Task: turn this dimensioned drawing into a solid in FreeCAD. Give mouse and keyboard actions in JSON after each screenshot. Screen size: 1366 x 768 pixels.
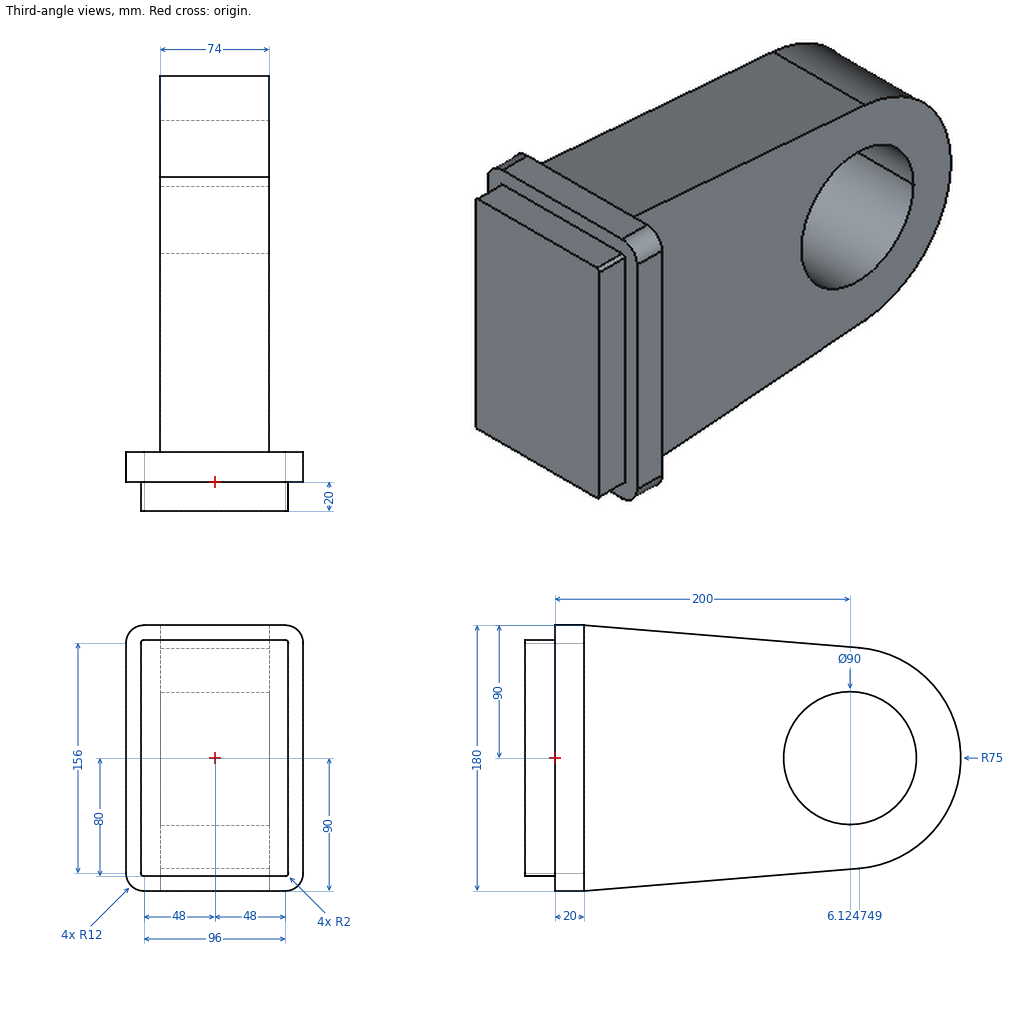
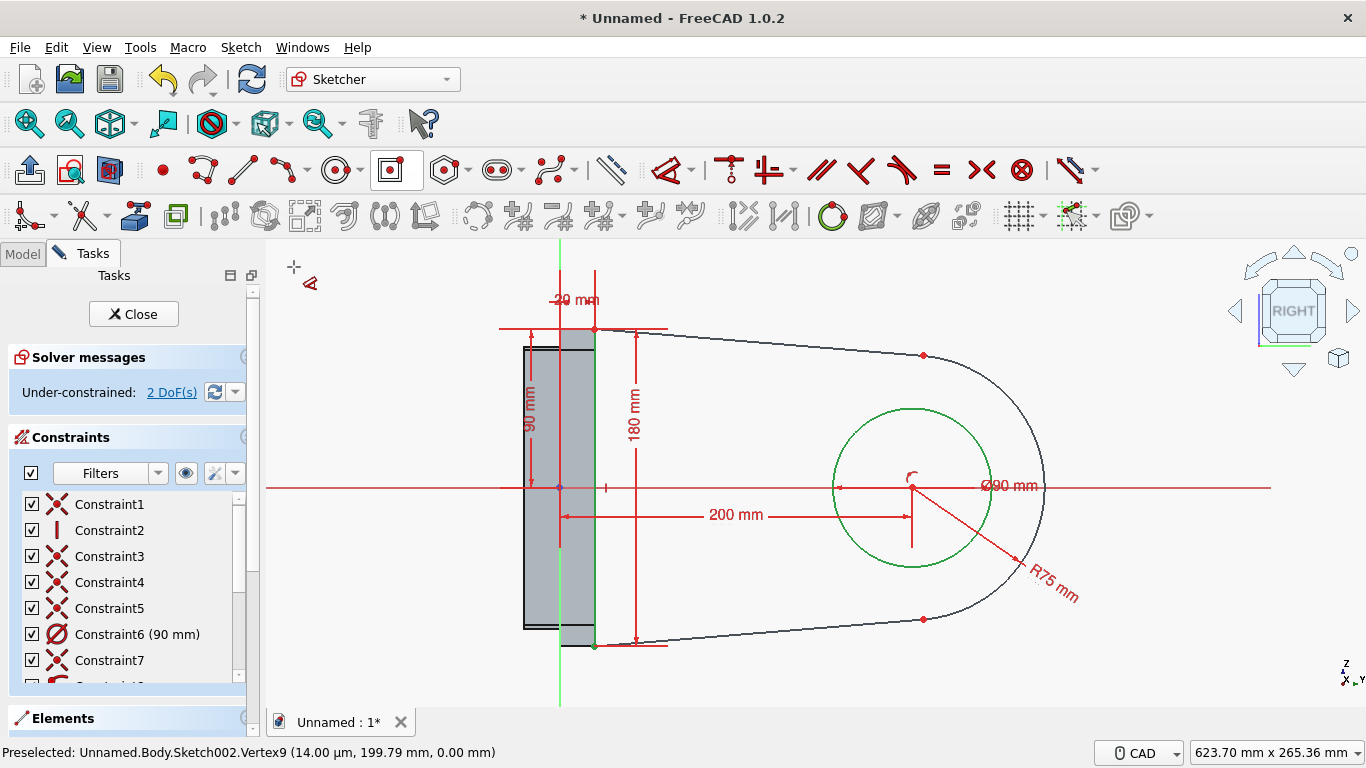
{"action": "scroll", "coordinate": [924, 620], "scroll_direction": "up", "scroll_amount": 7}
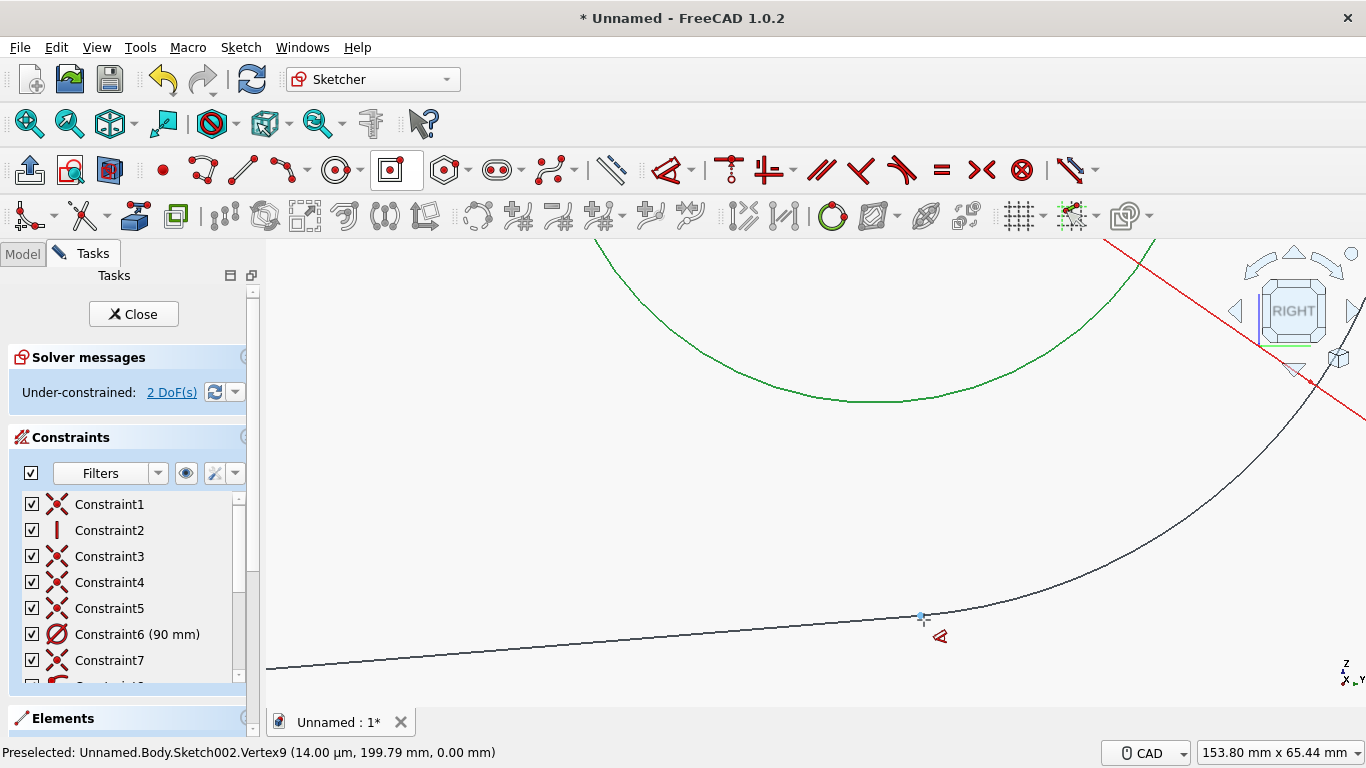
{"action": "left_click", "coordinate": [921, 616]}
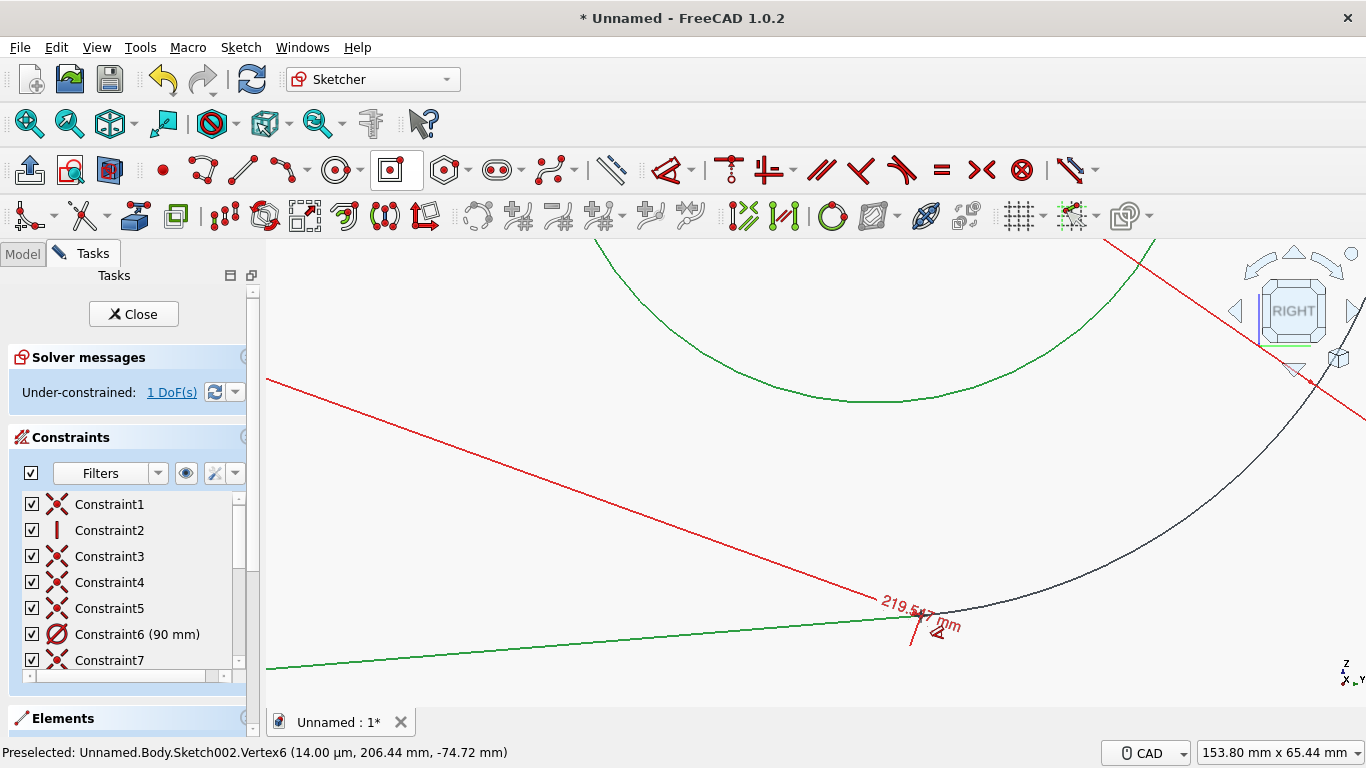
{"action": "scroll", "coordinate": [852, 601], "scroll_direction": "down", "scroll_amount": 7}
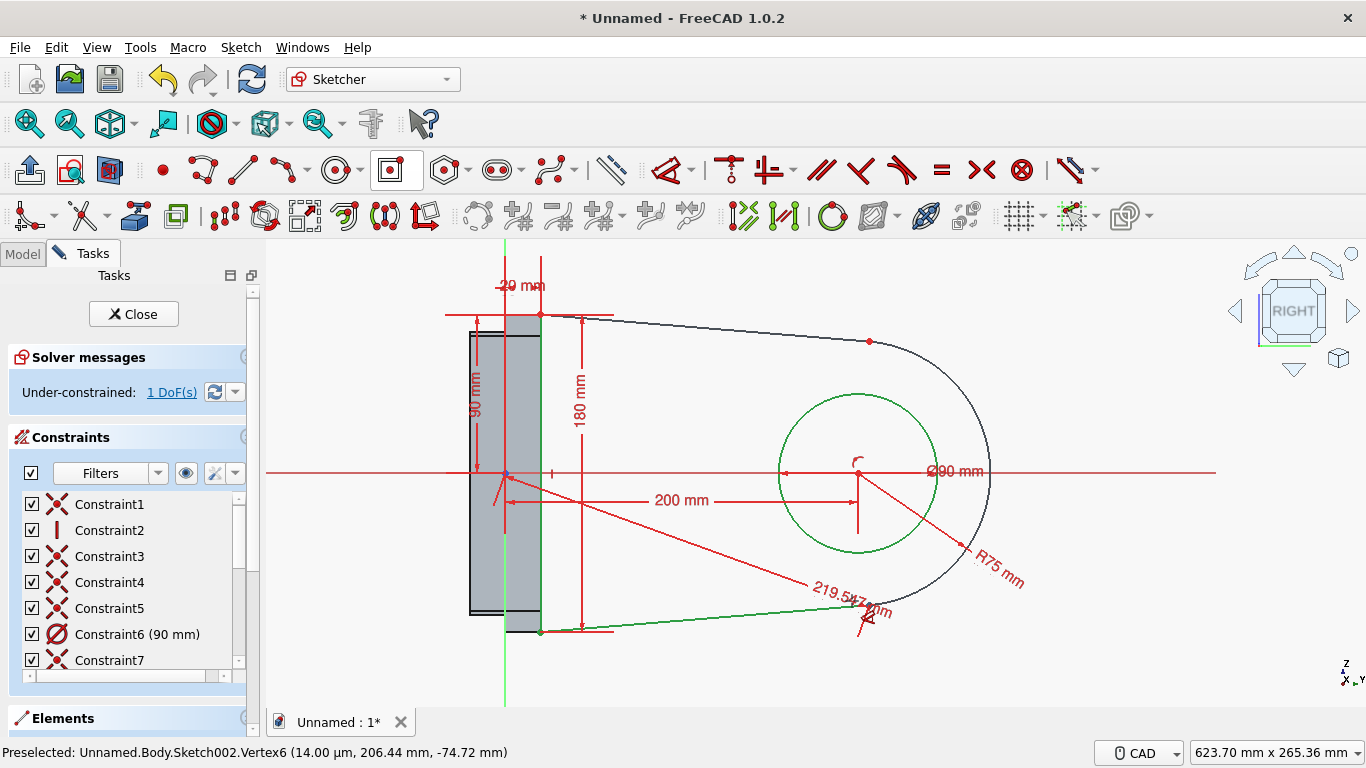
{"action": "scroll", "coordinate": [858, 473], "scroll_direction": "up", "scroll_amount": 7}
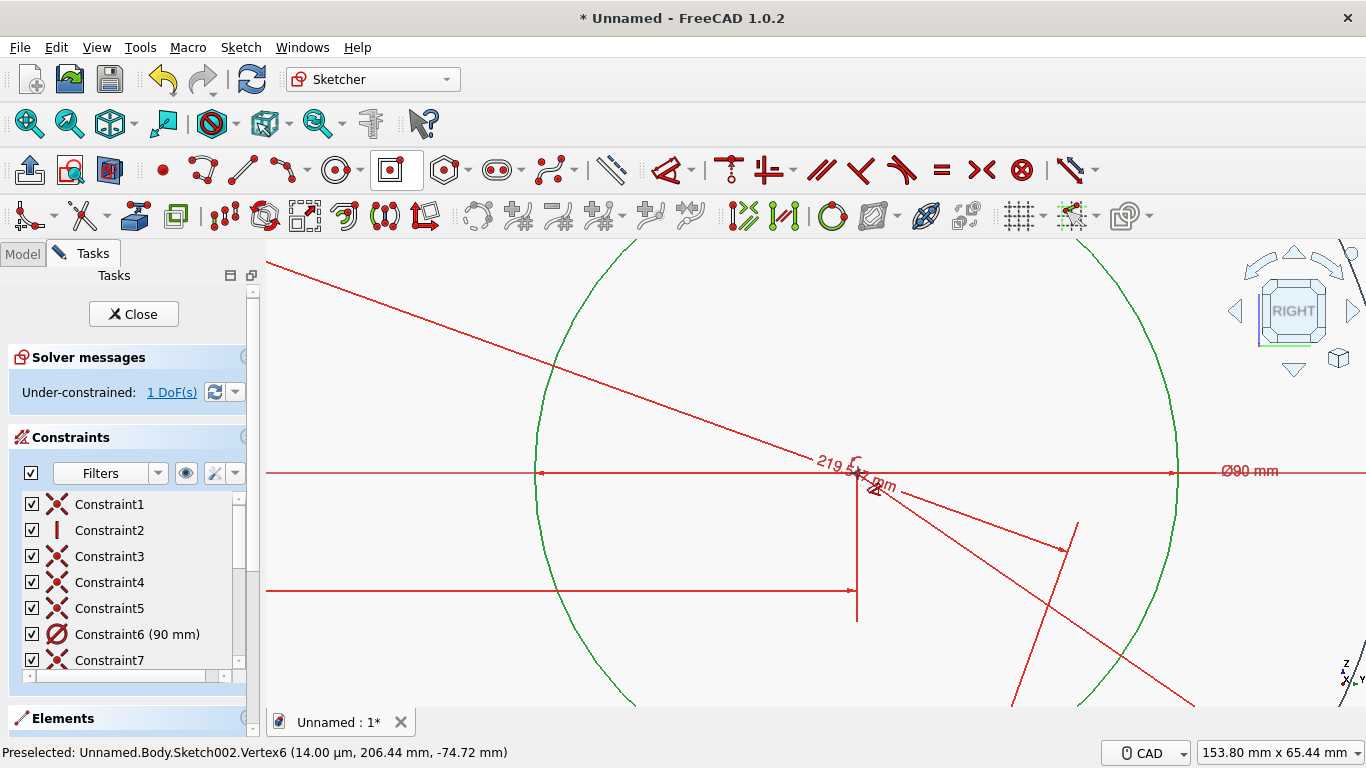
{"action": "left_click", "coordinate": [857, 473]}
{"action": "left_click", "coordinate": [880, 439]}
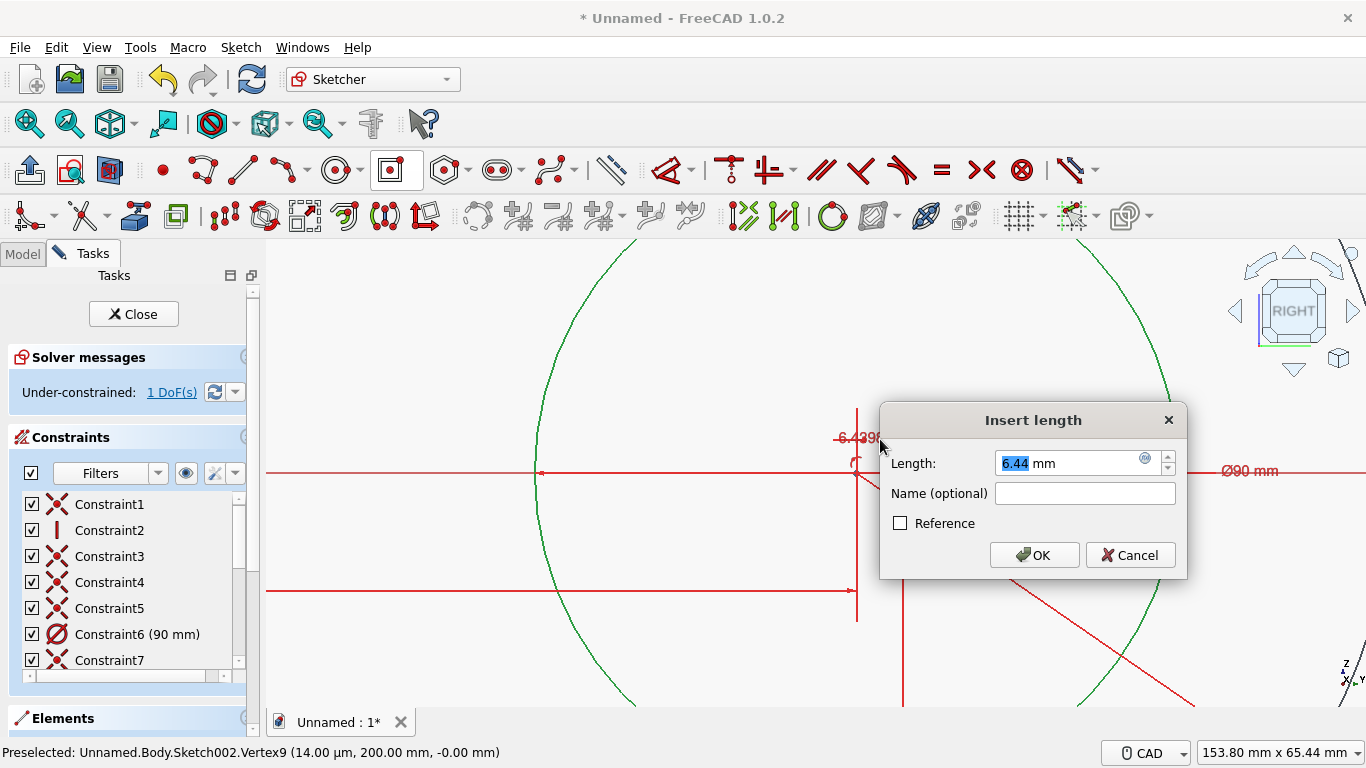
{"action": "type", "text": "6.124749"}
{"action": "key", "text": "Return"}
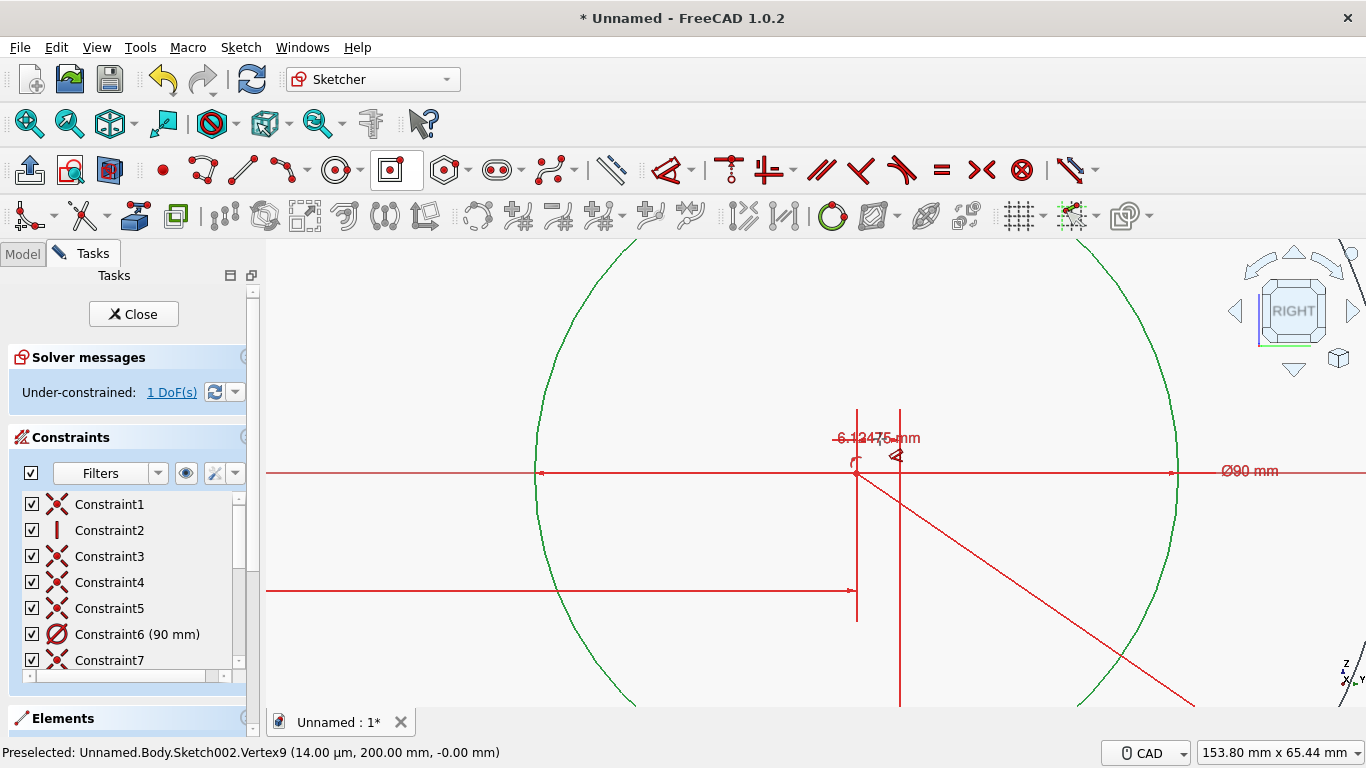
{"action": "scroll", "coordinate": [858, 473], "scroll_direction": "down", "scroll_amount": 7}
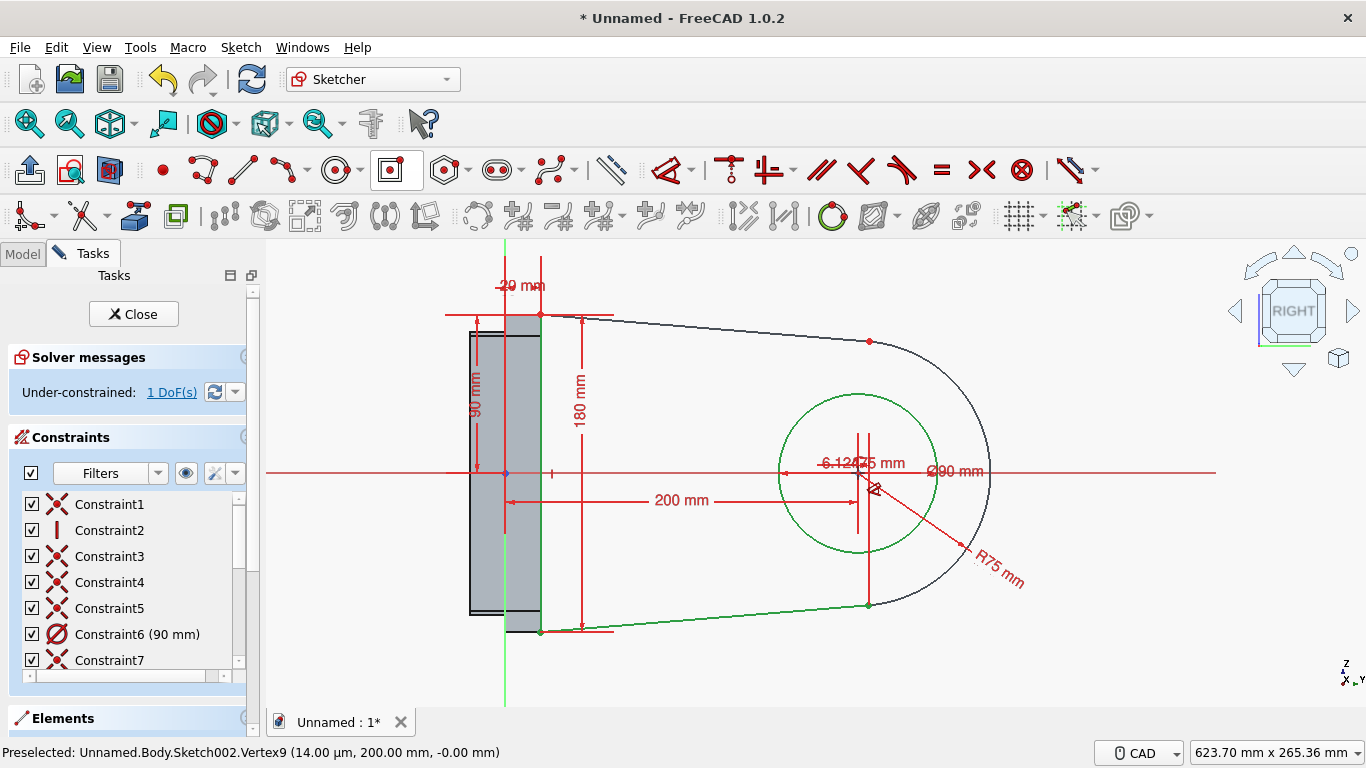
{"action": "scroll", "coordinate": [869, 342], "scroll_direction": "up", "scroll_amount": 7}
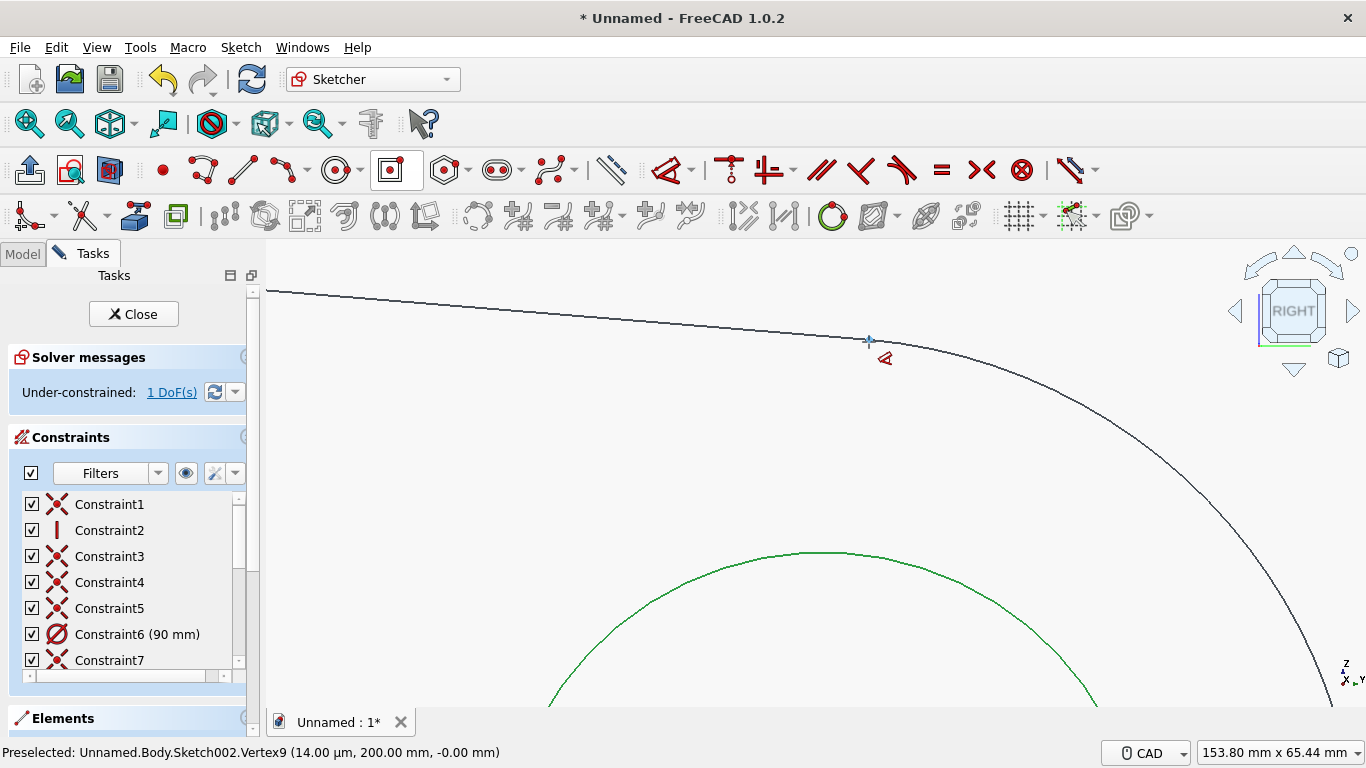
{"action": "left_click", "coordinate": [869, 340]}